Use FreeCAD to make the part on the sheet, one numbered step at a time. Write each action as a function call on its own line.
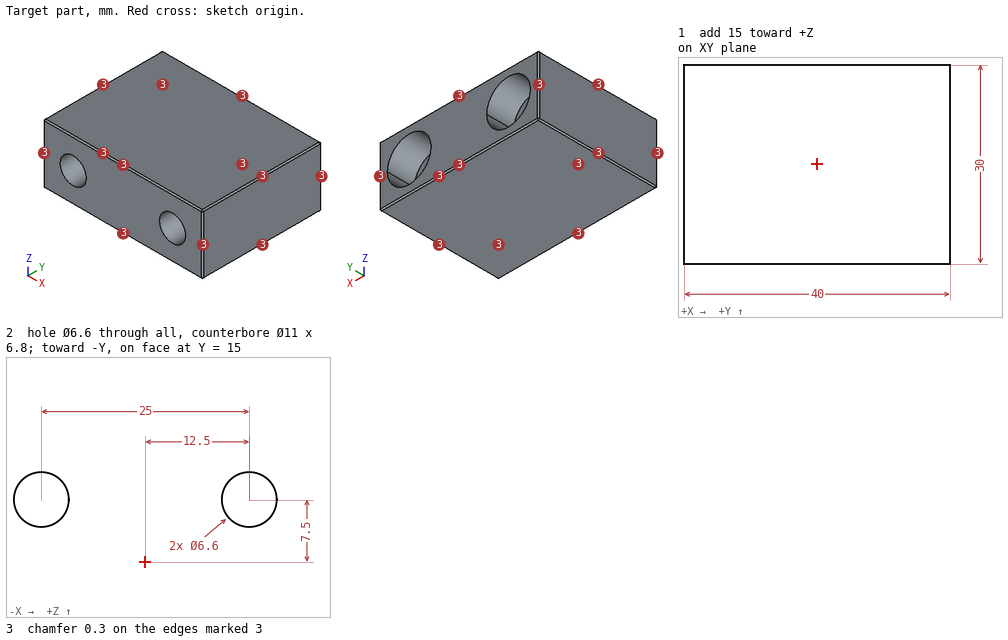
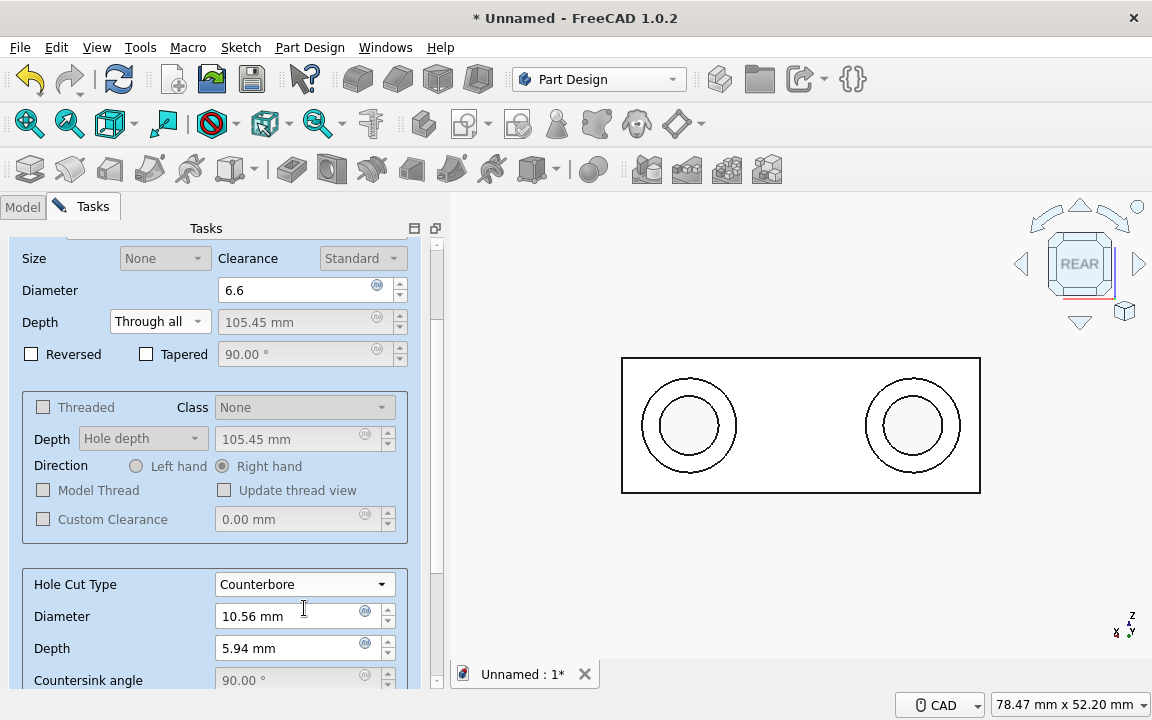
triple_click(298, 616)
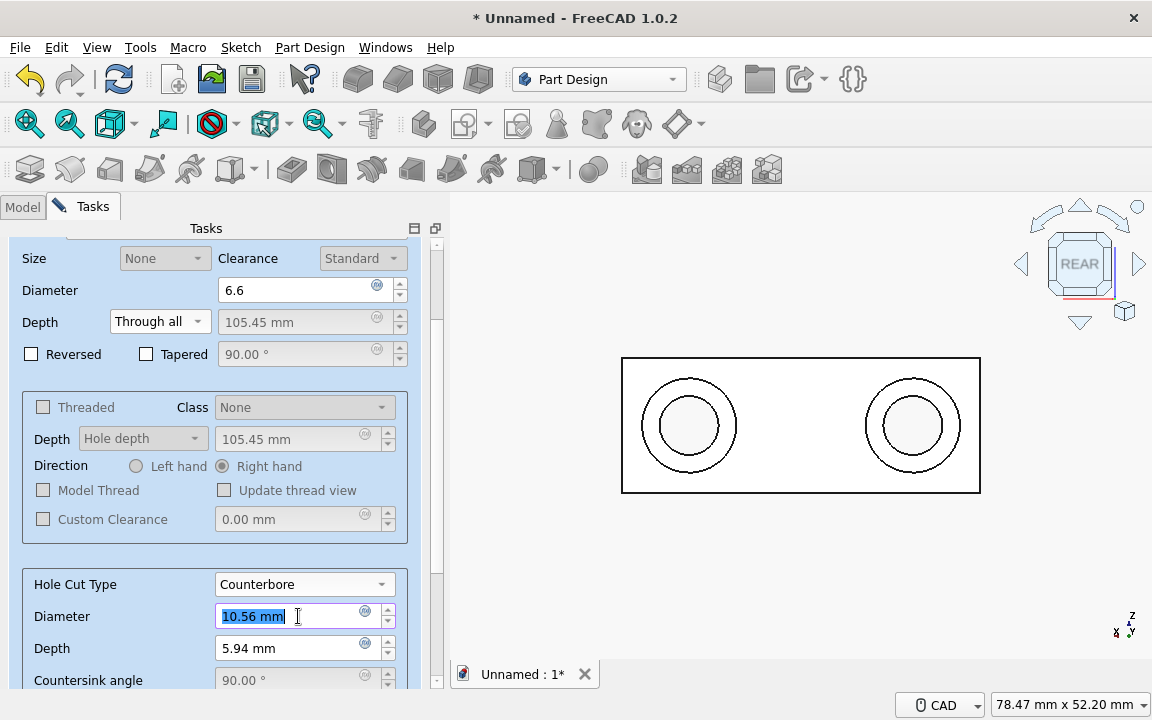
text(11)
key(Tab)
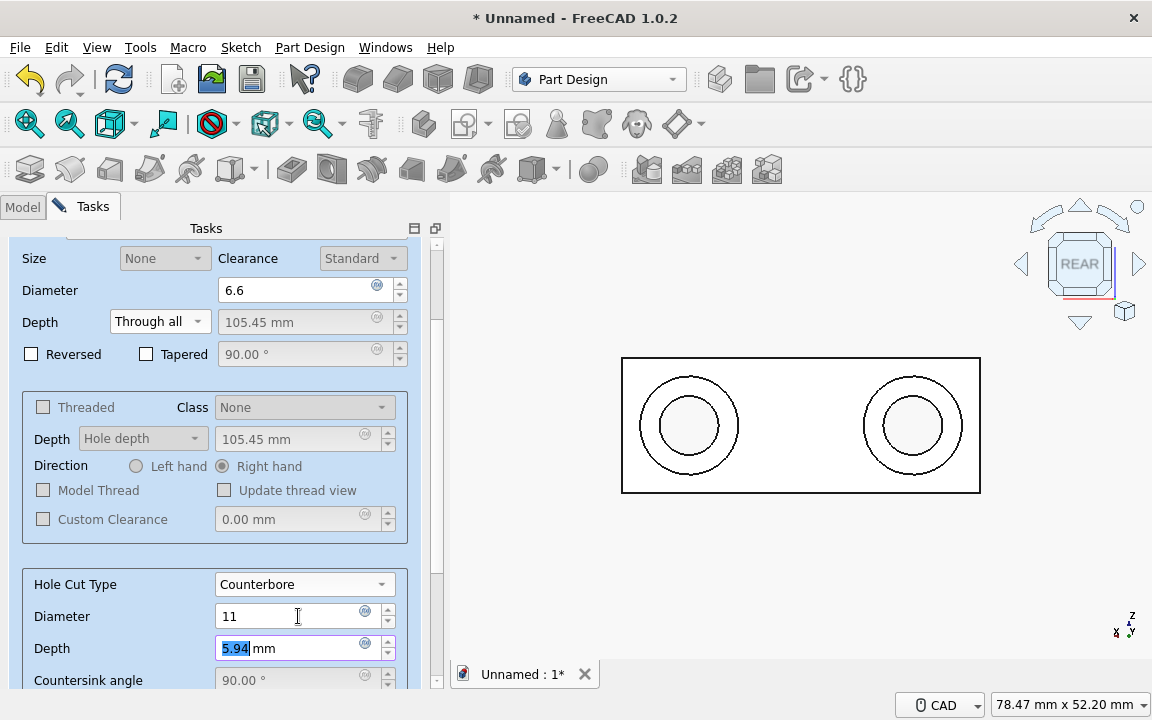
text(6.8)
key(Tab)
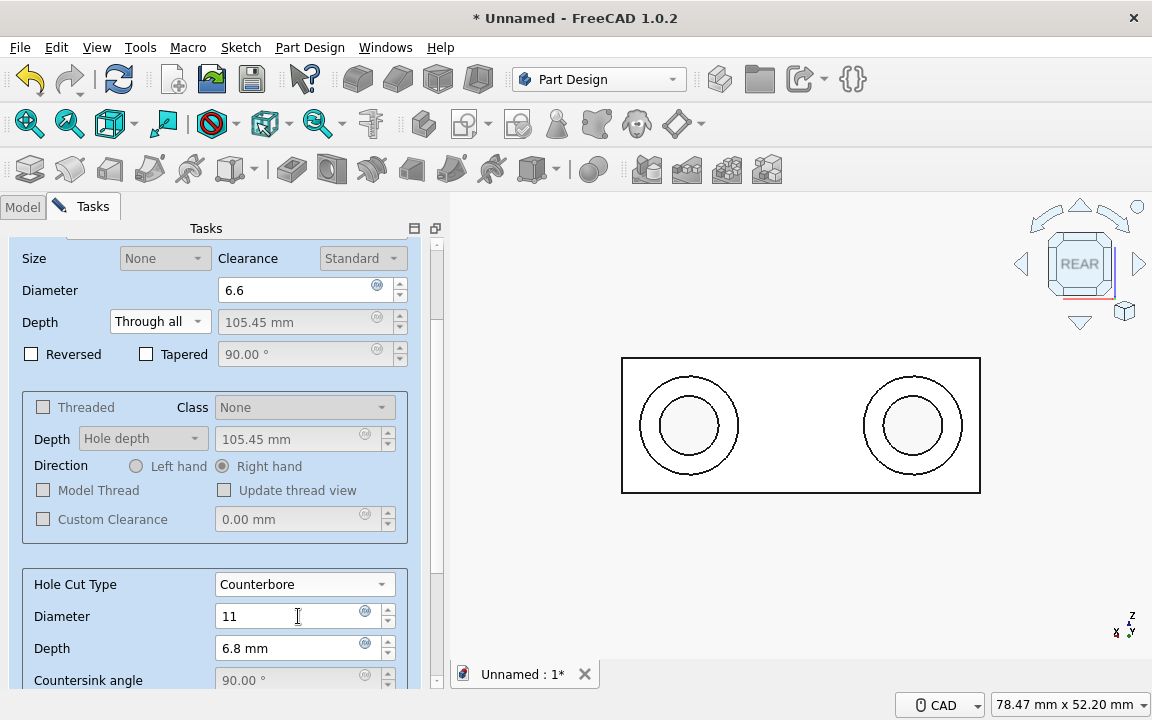
scroll(437, 463, up, 3)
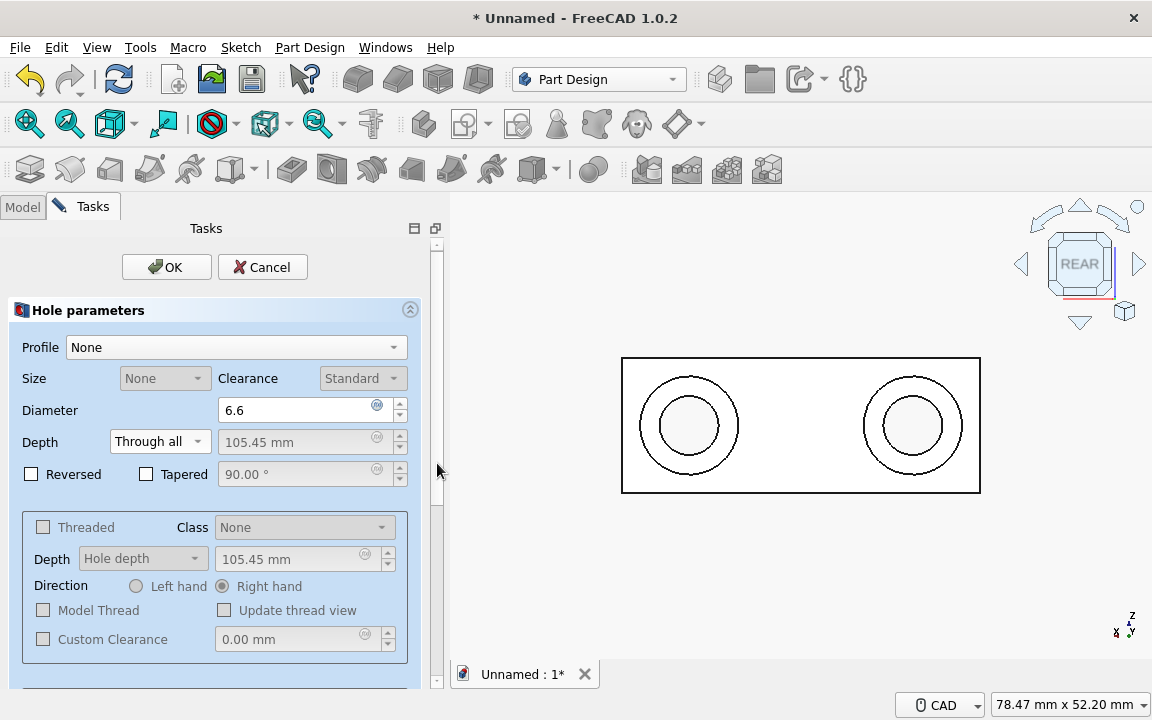
click(167, 267)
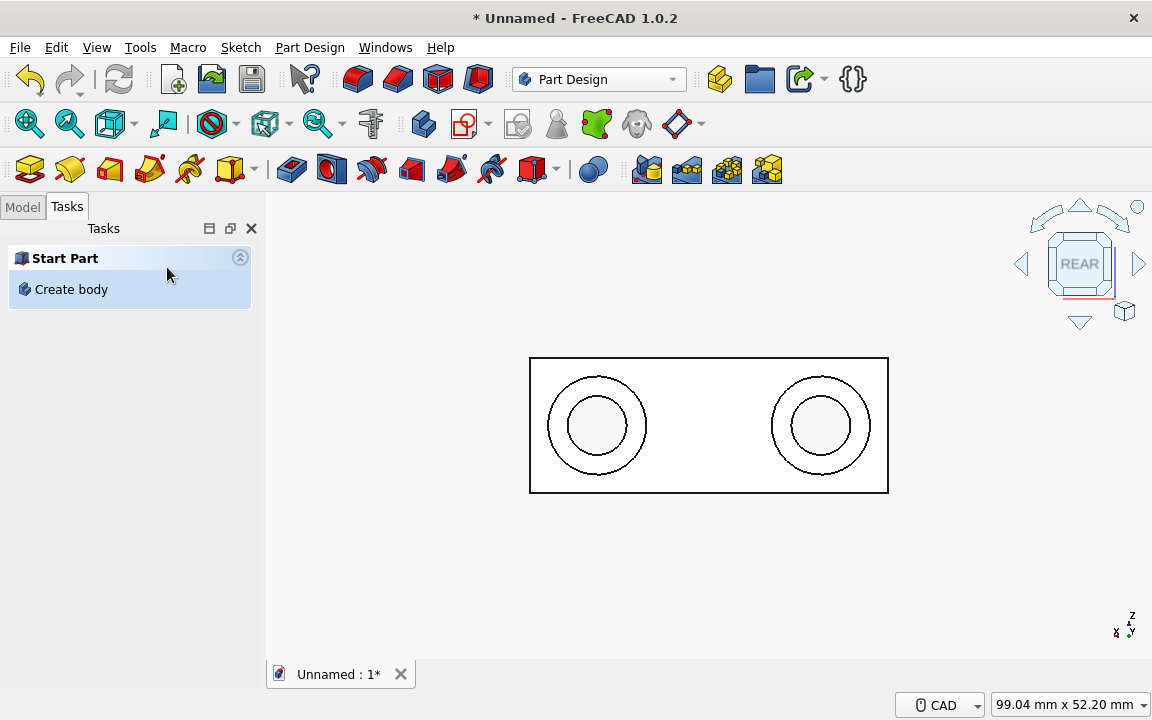
key(v)
key(f)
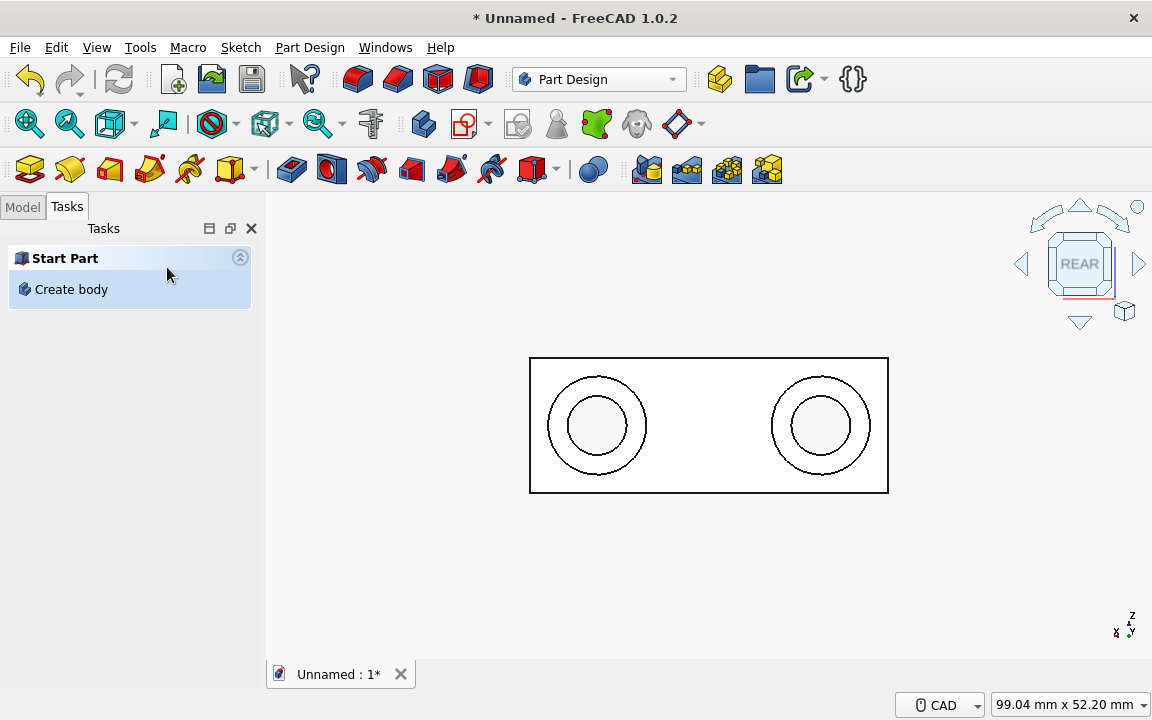
click(888, 424)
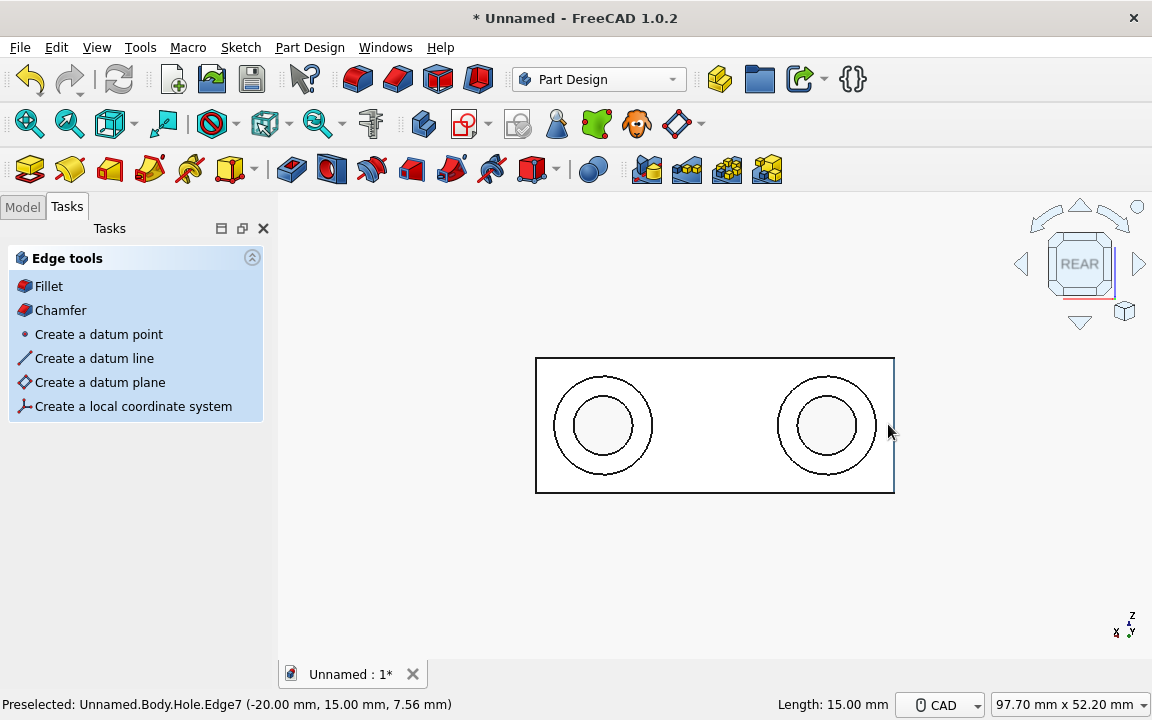
key(0)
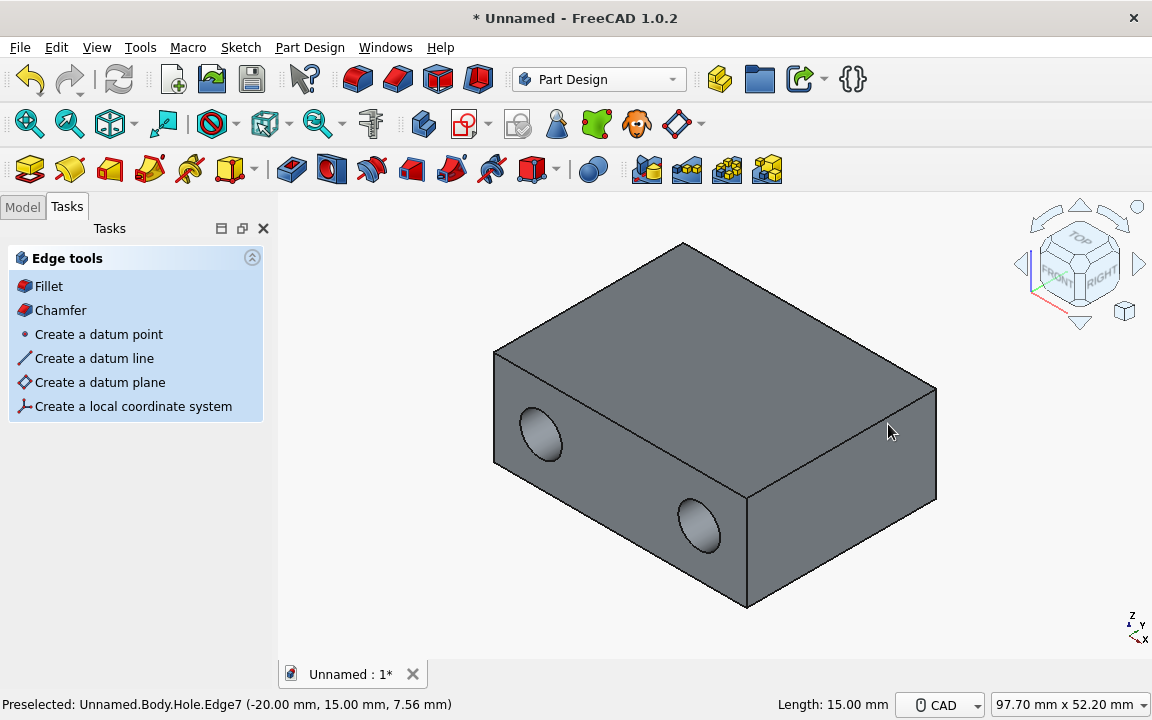
click(715, 370, ctrl)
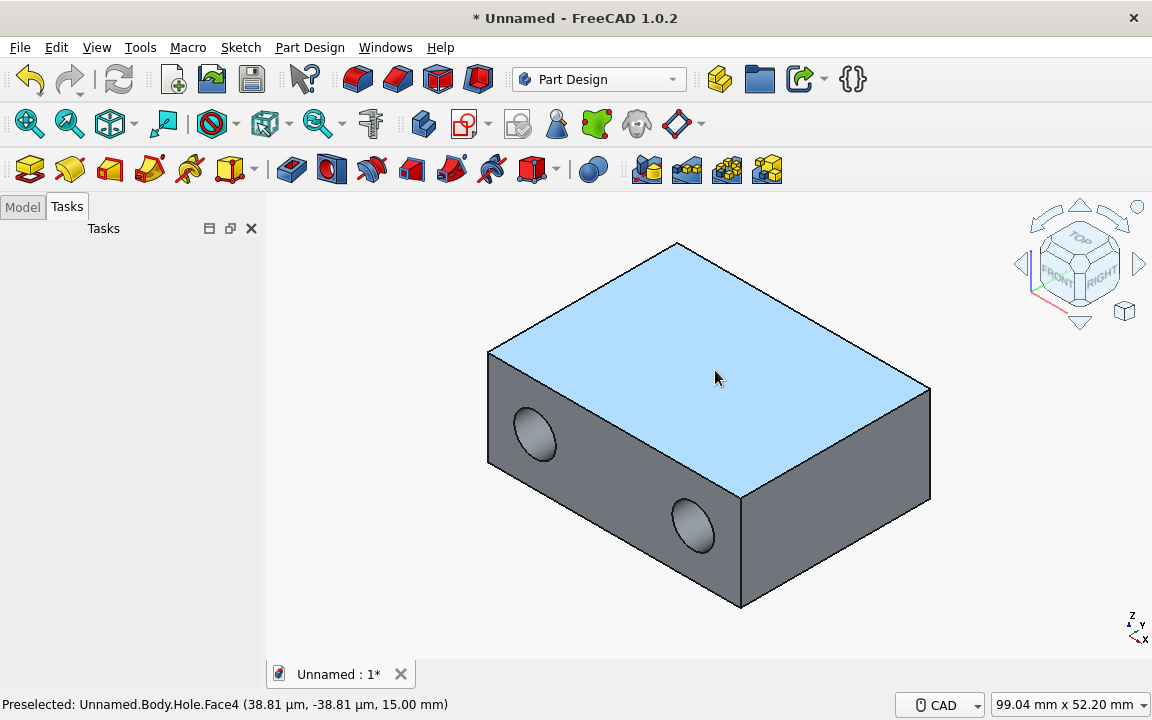
click(741, 552, ctrl)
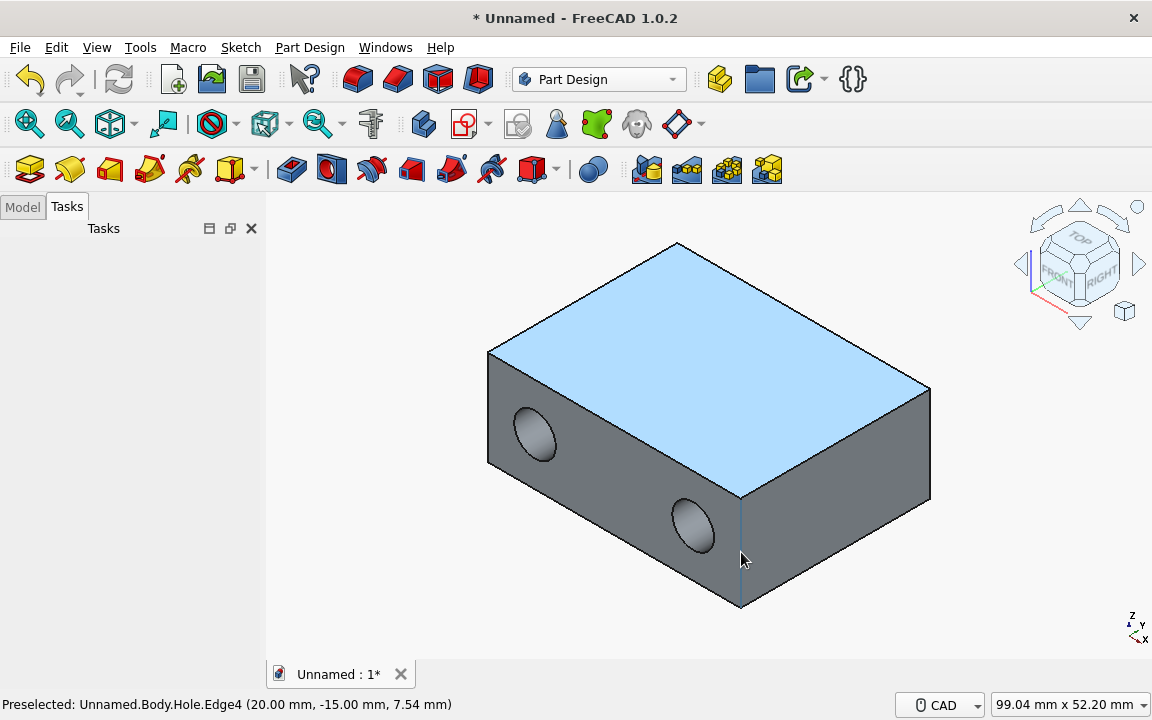
key(2)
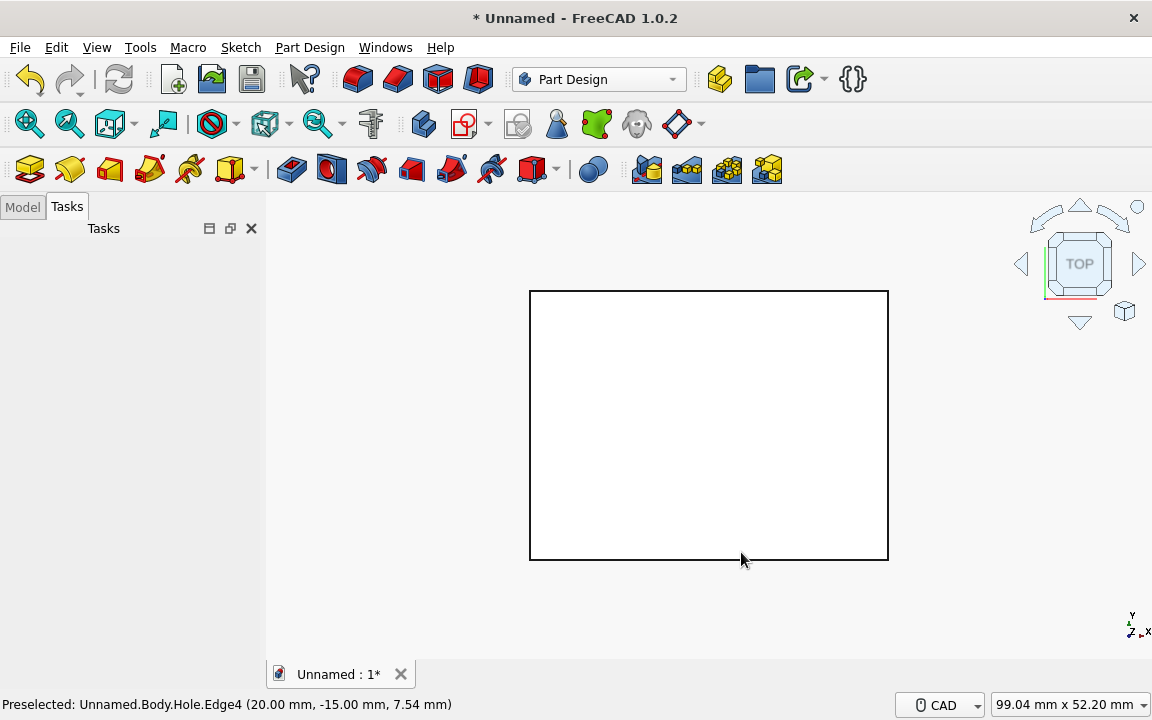
key(1)